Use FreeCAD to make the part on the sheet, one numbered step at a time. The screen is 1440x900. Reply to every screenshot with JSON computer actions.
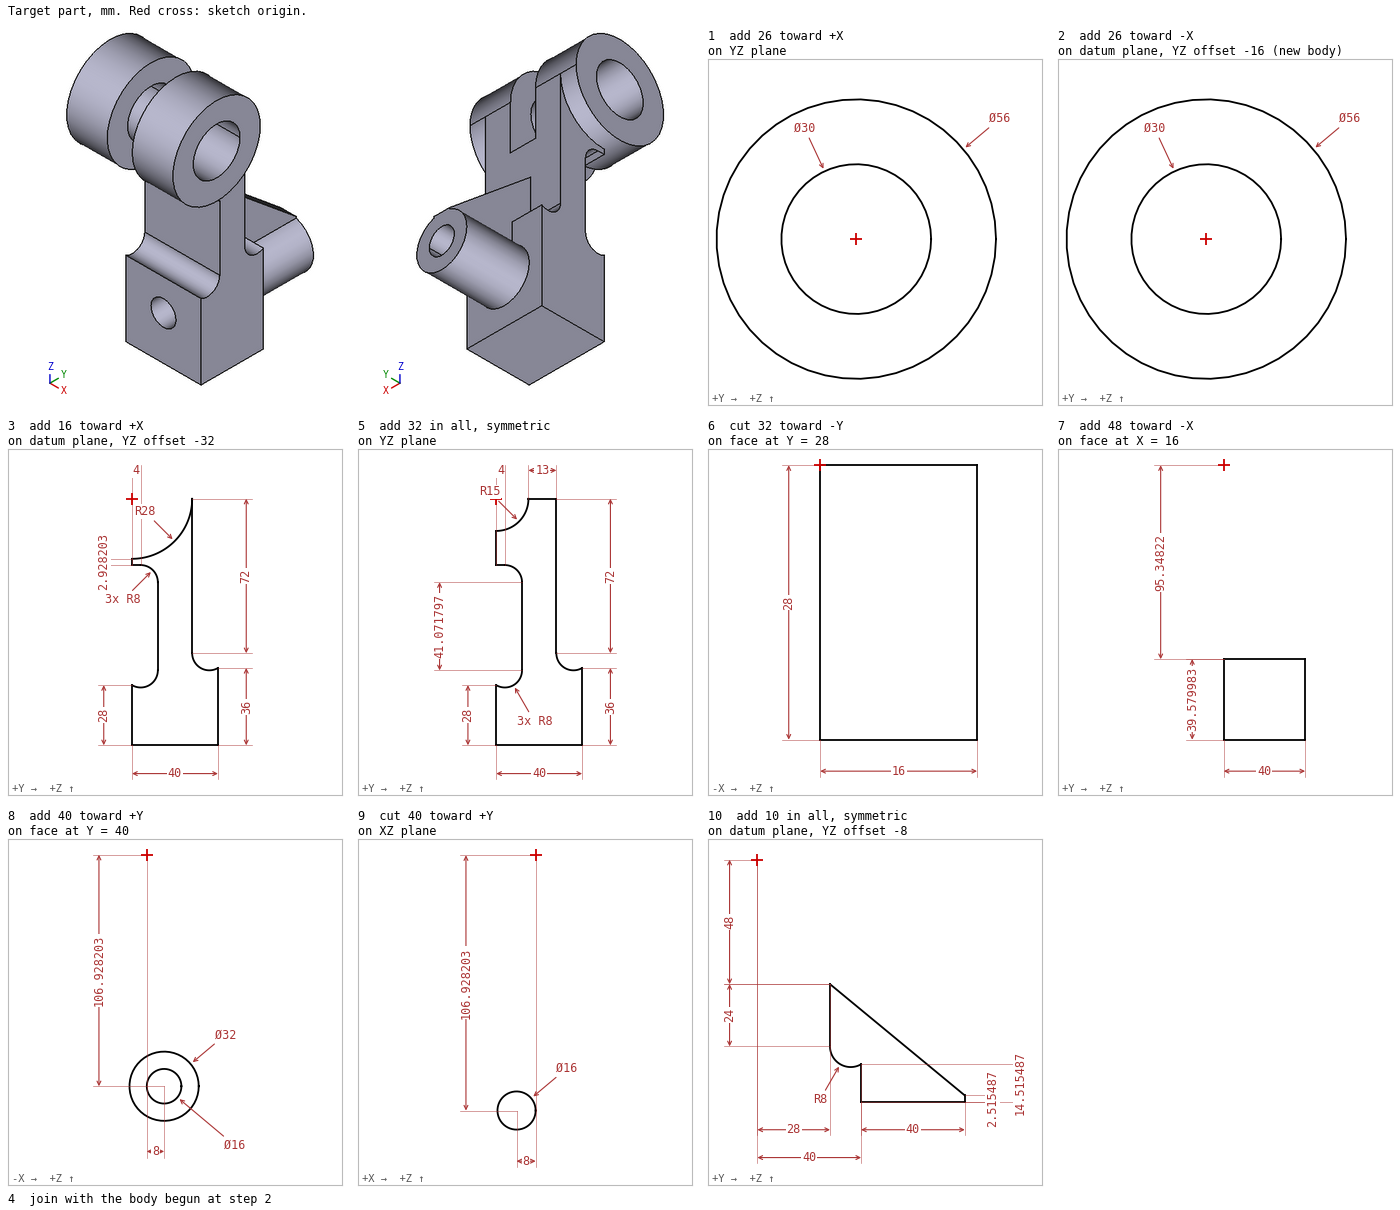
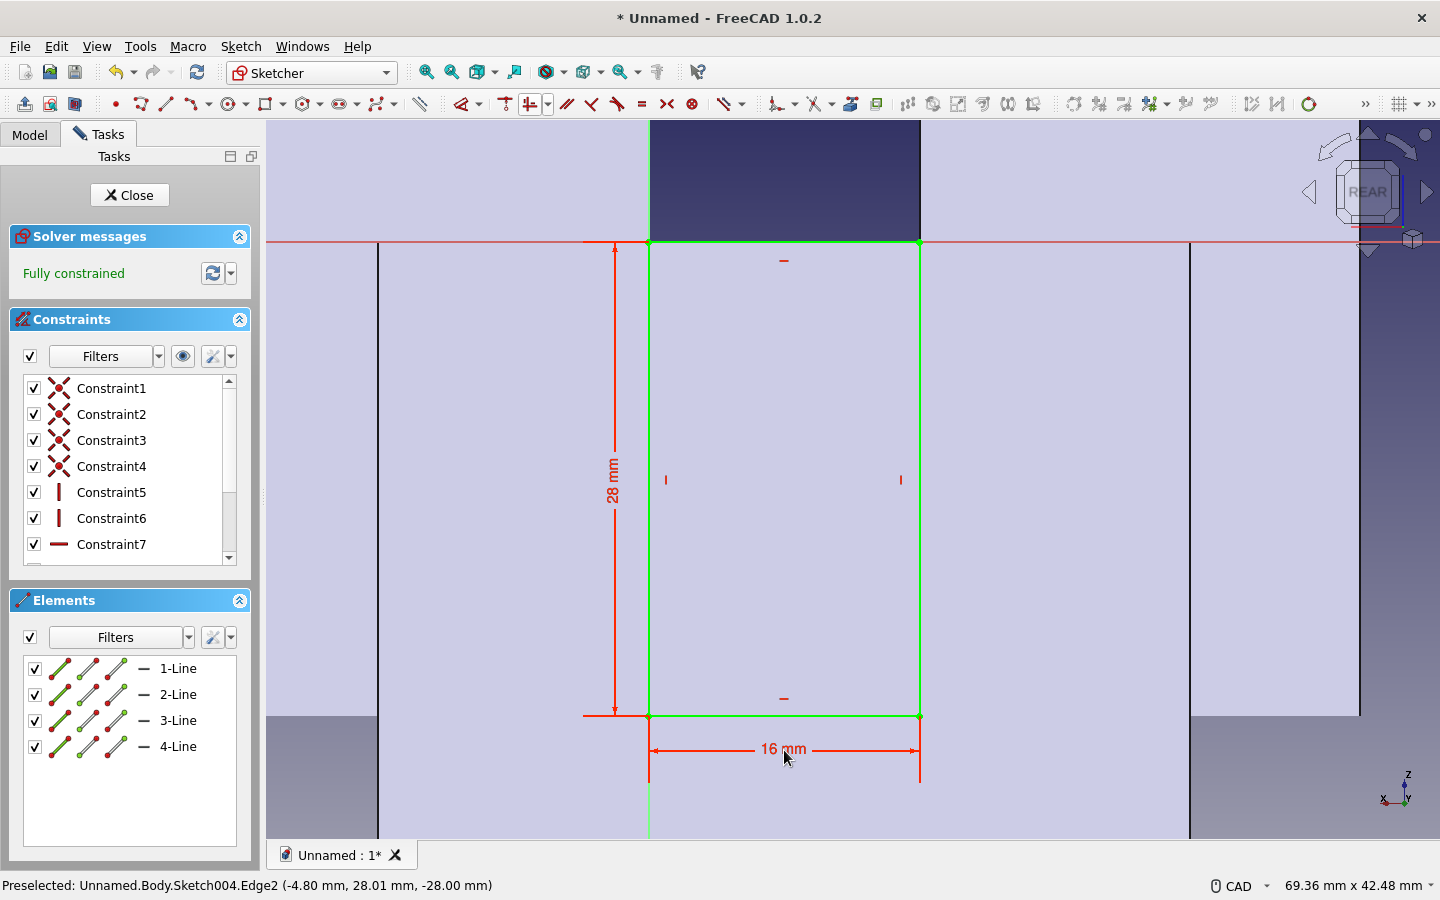
{"action": "left_click", "coordinate": [130, 195]}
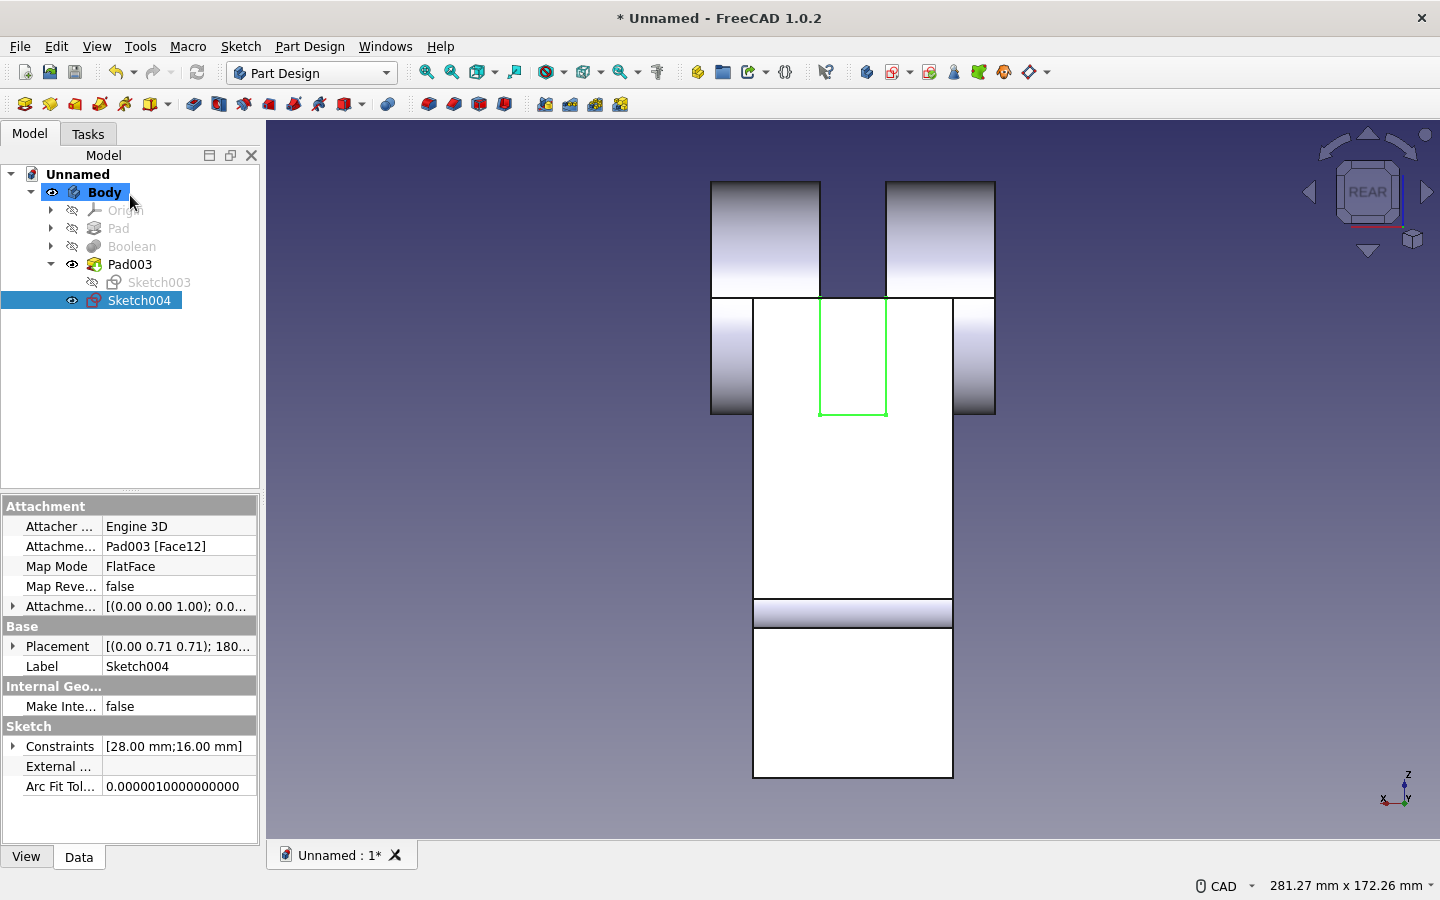
{"action": "left_click", "coordinate": [194, 104]}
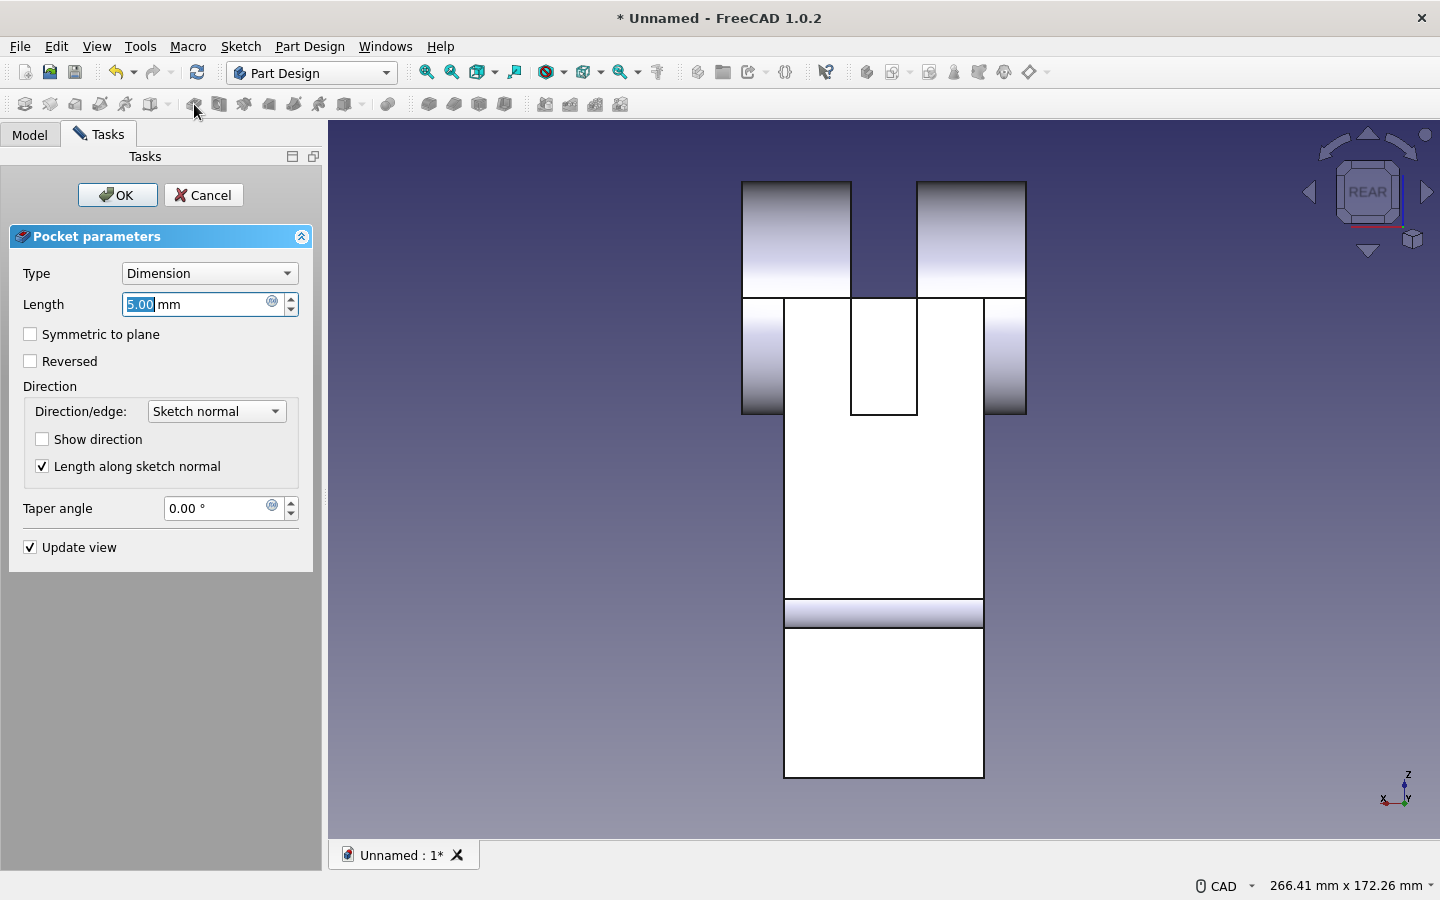
{"action": "type", "text": "32"}
{"action": "key", "text": "Tab"}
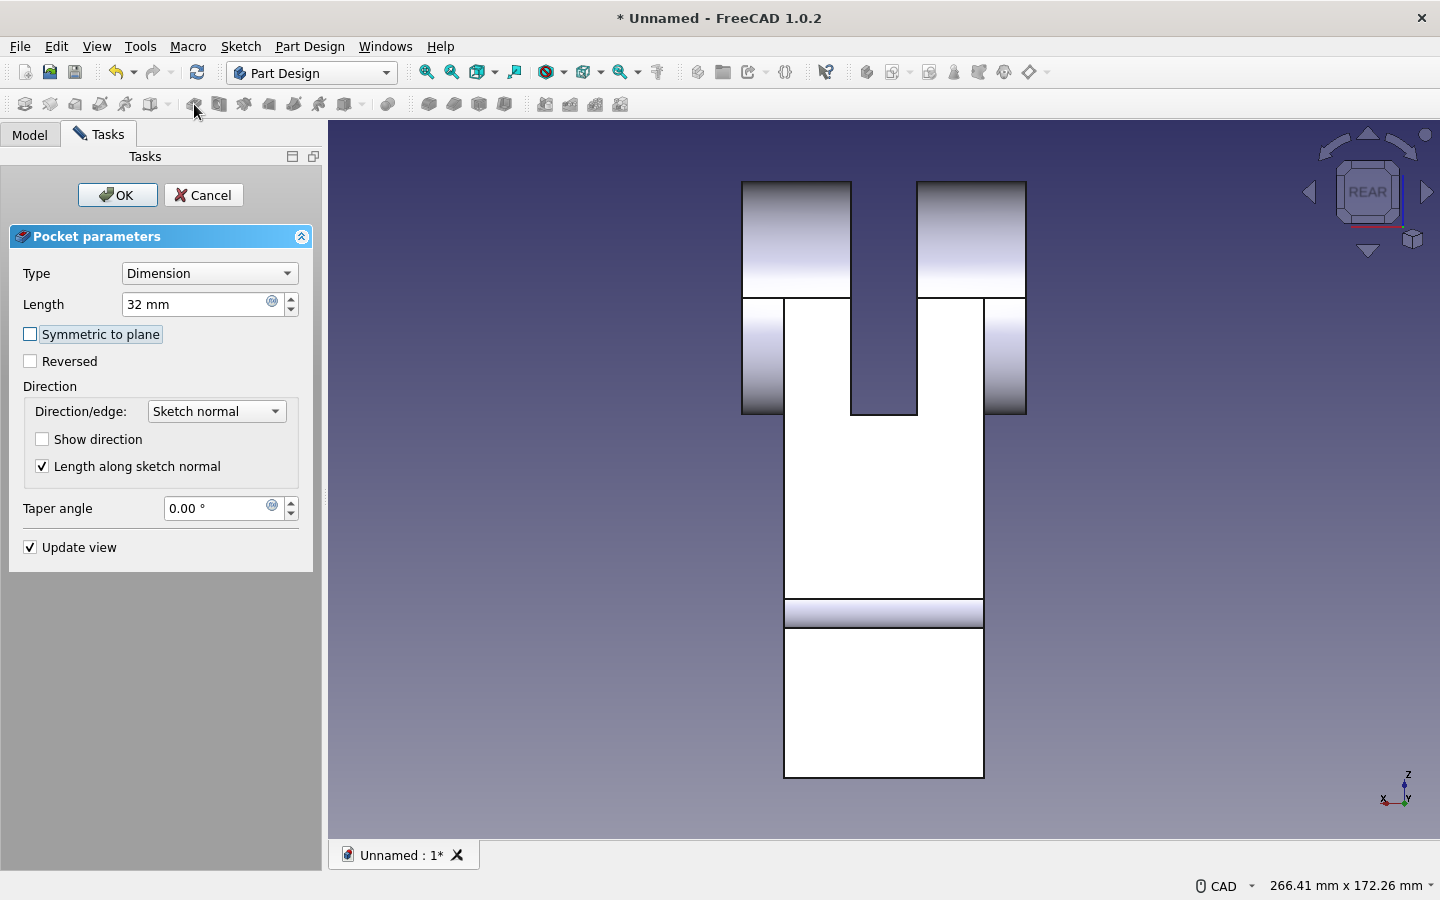
{"action": "left_click", "coordinate": [118, 195]}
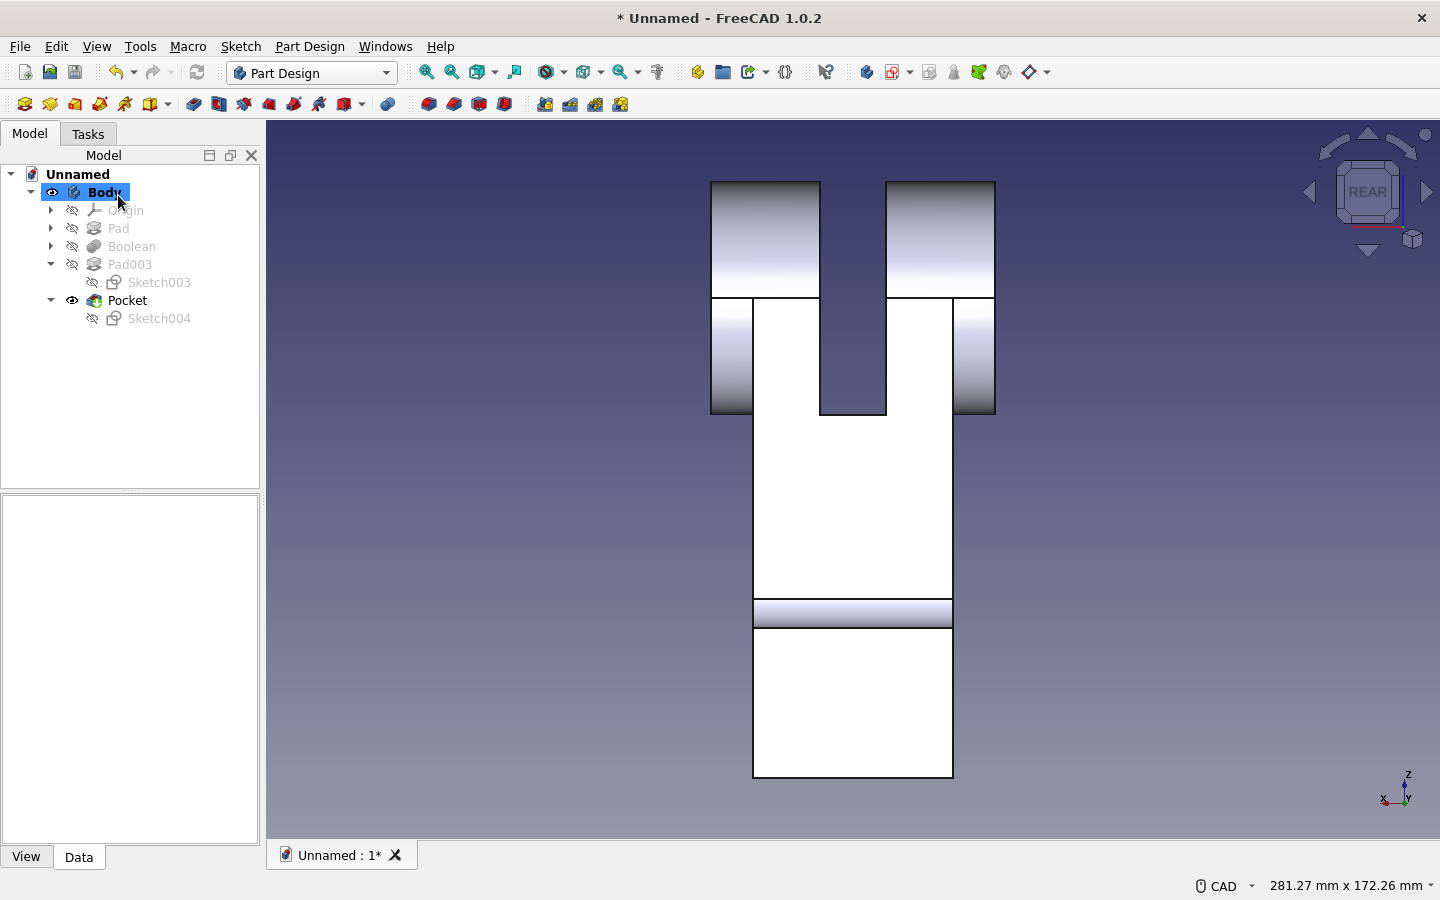
{"action": "key", "text": "0"}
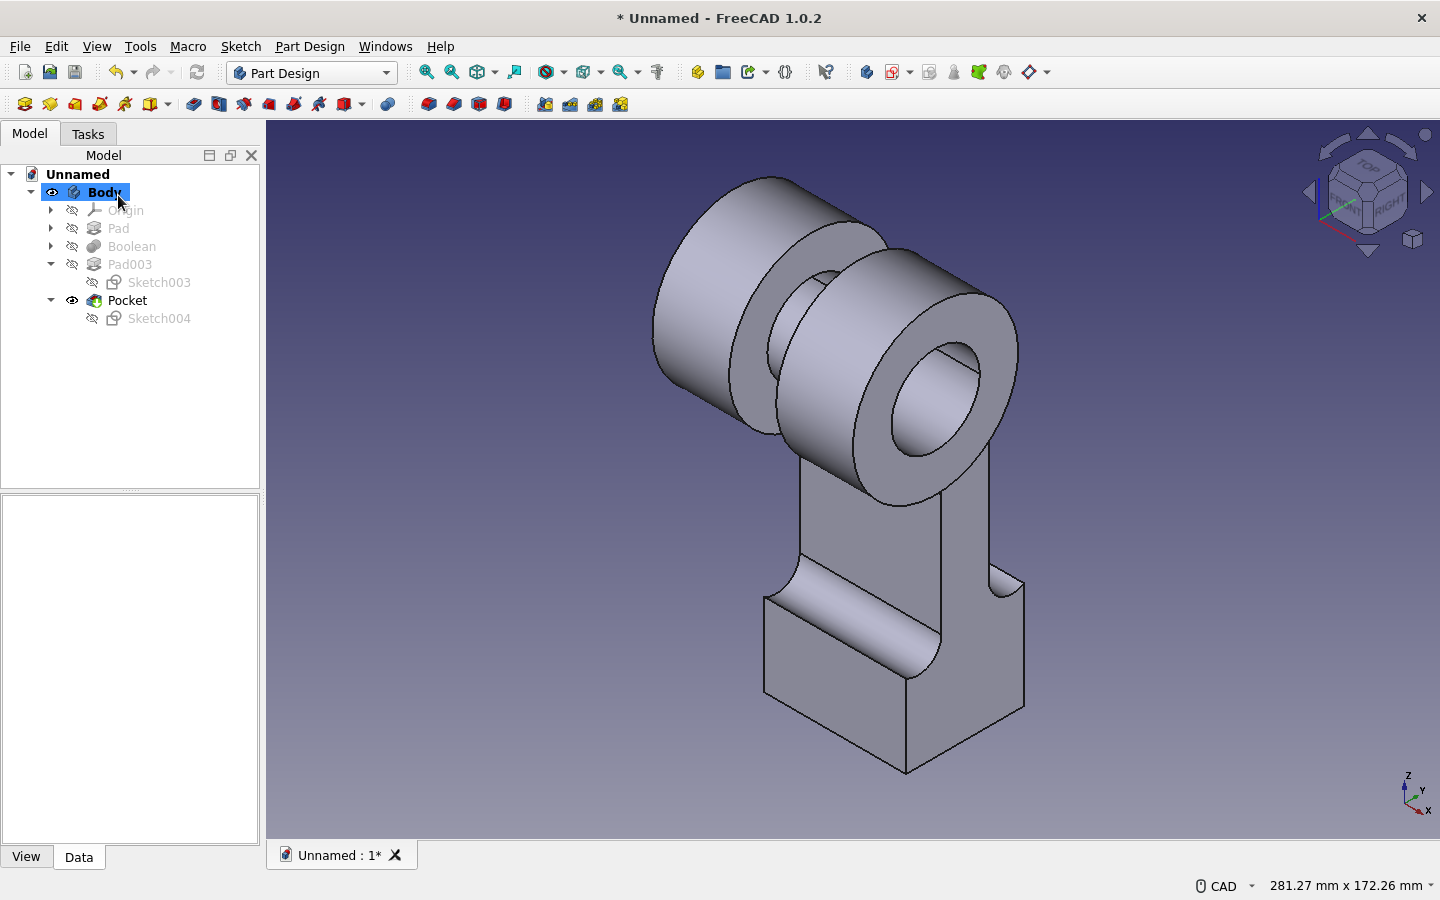
{"action": "key", "text": "v f"}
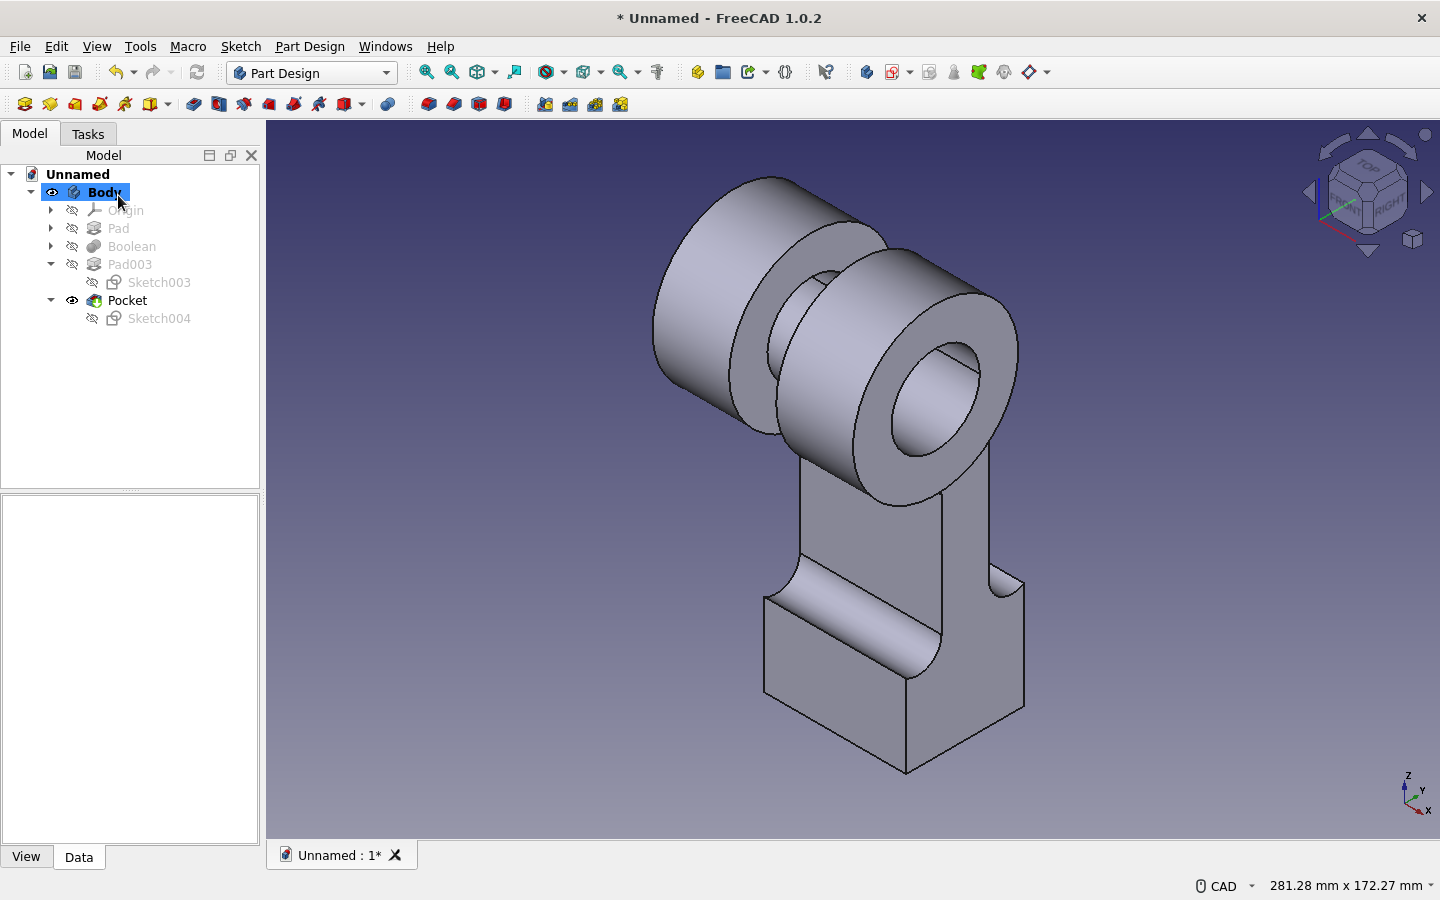
{"action": "left_click", "coordinate": [982, 645]}